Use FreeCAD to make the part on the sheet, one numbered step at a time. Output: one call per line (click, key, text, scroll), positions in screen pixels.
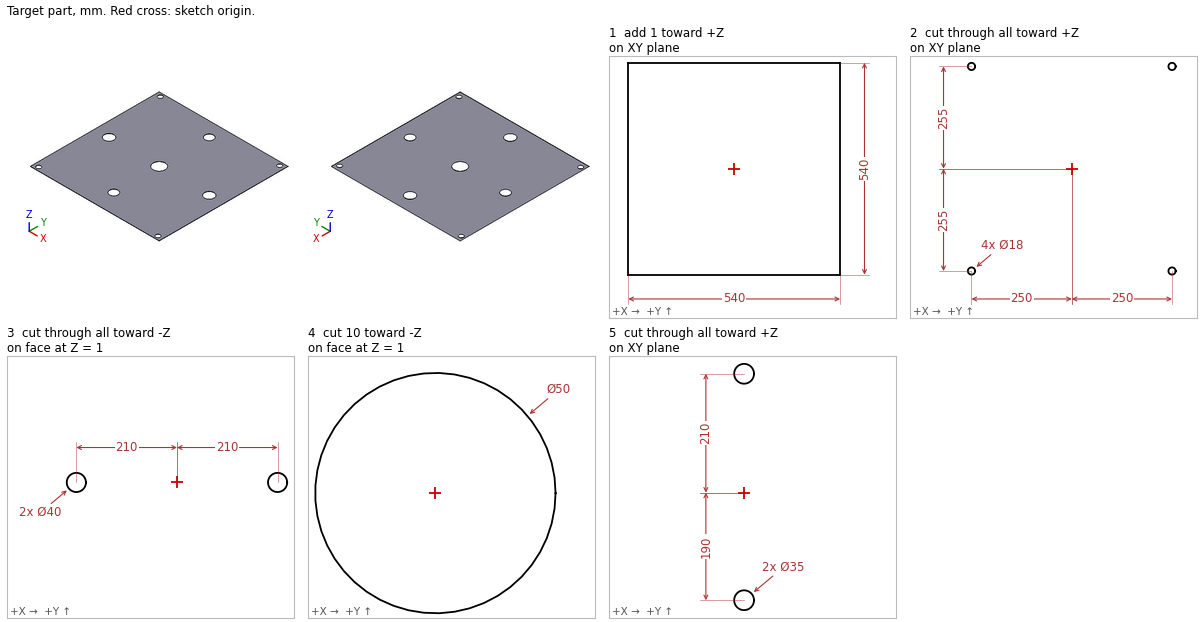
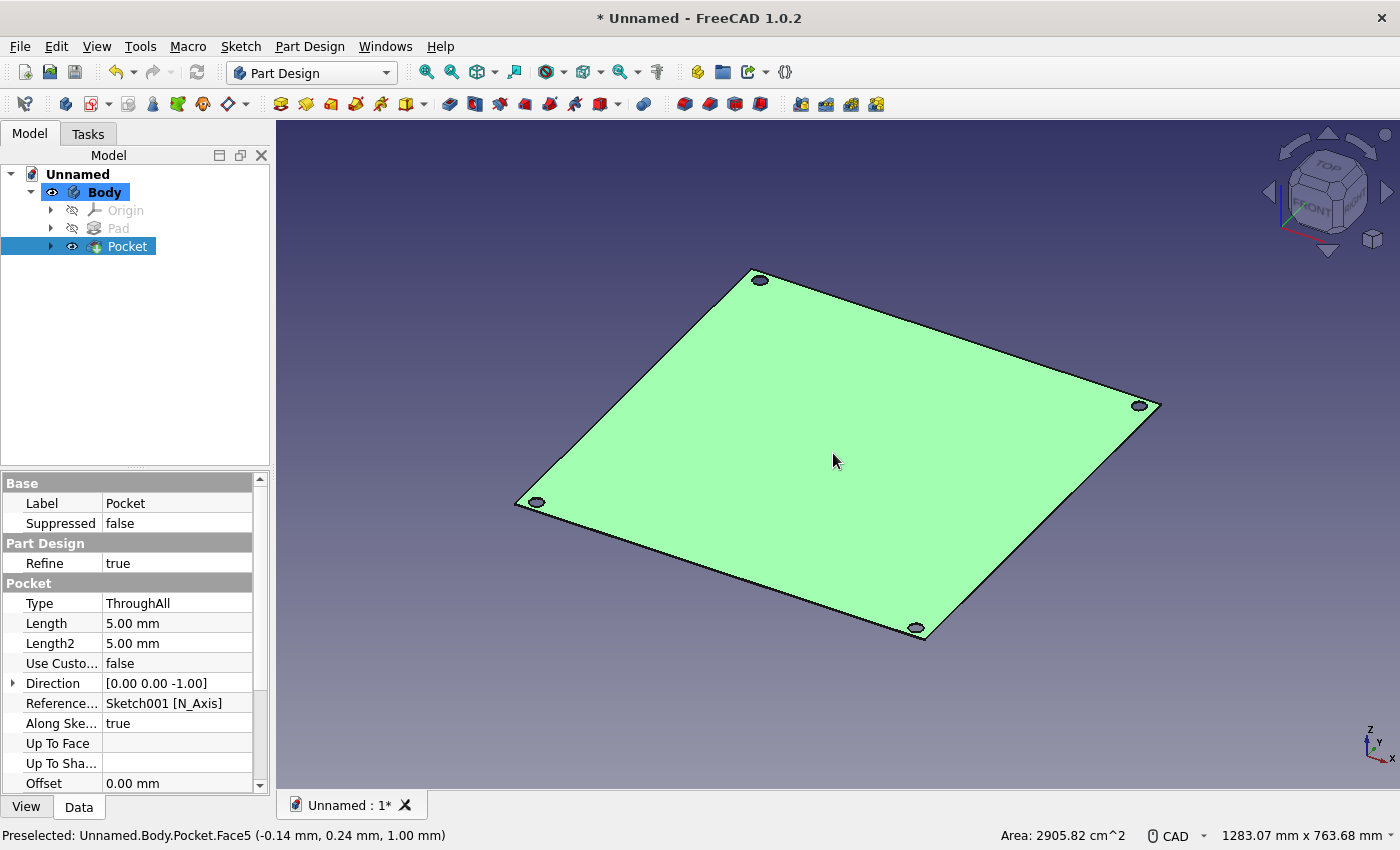
click(90, 104)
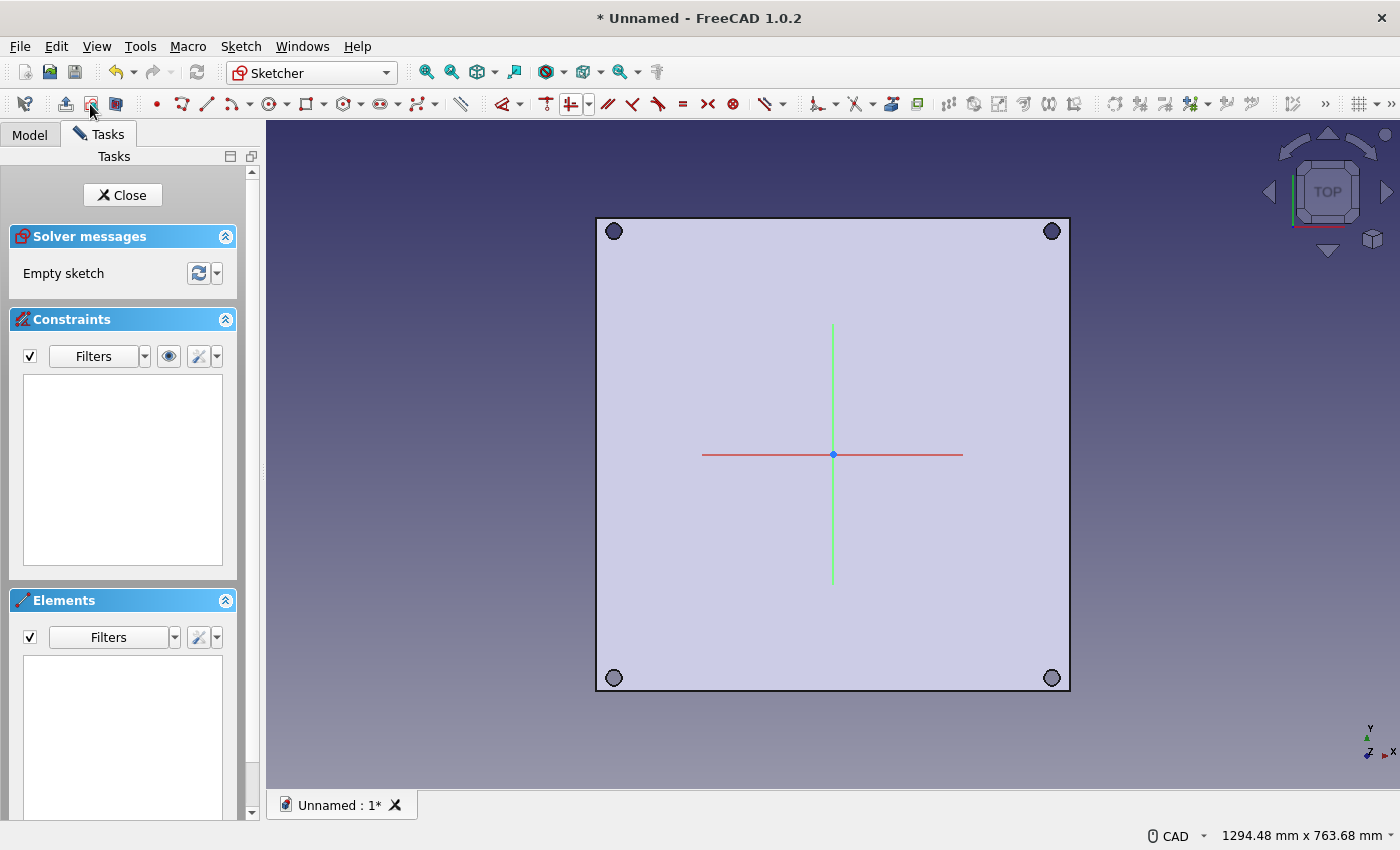
scroll(972, 455, up, 2)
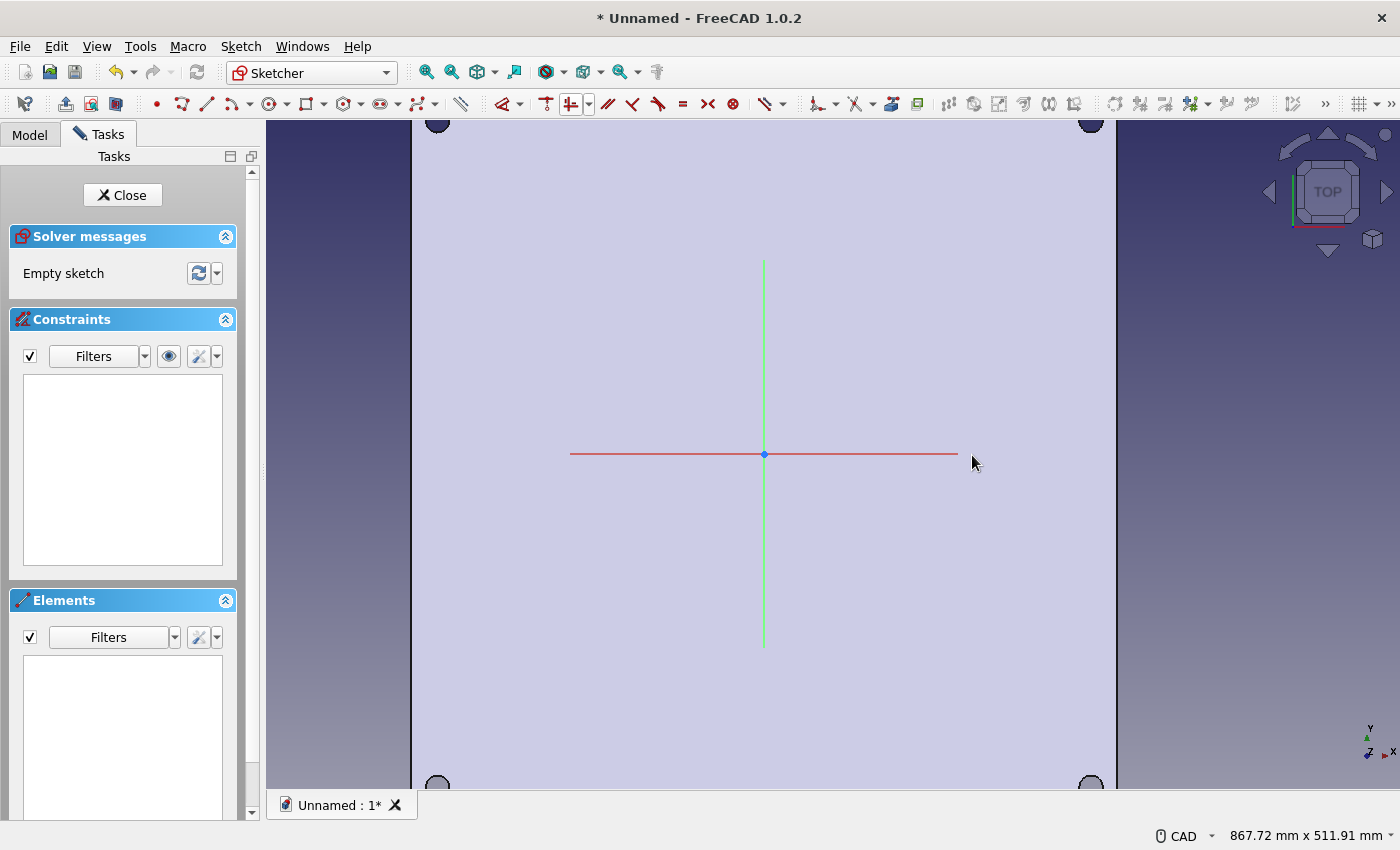
key(g)
key(c)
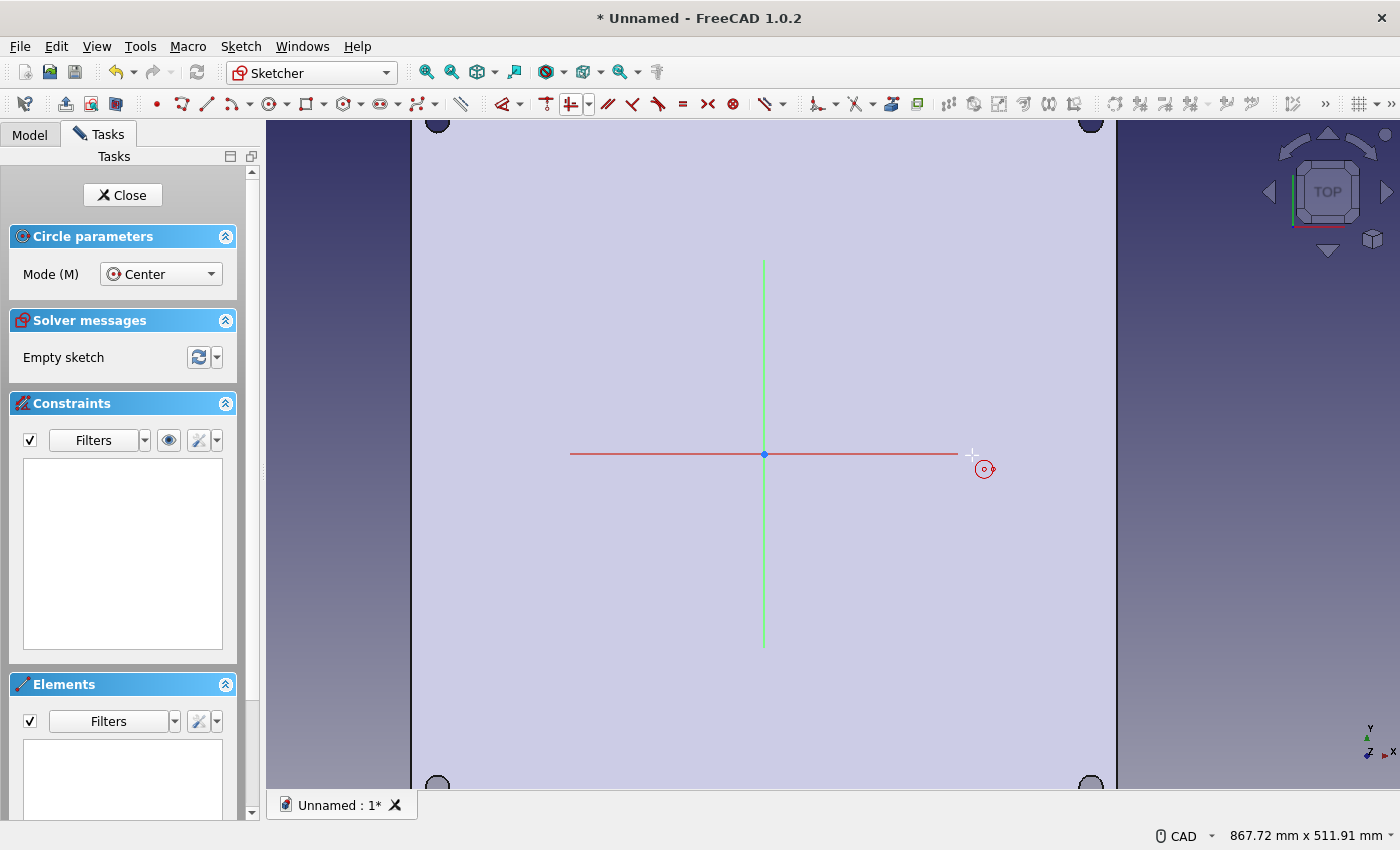
click(490, 454)
move(508, 436)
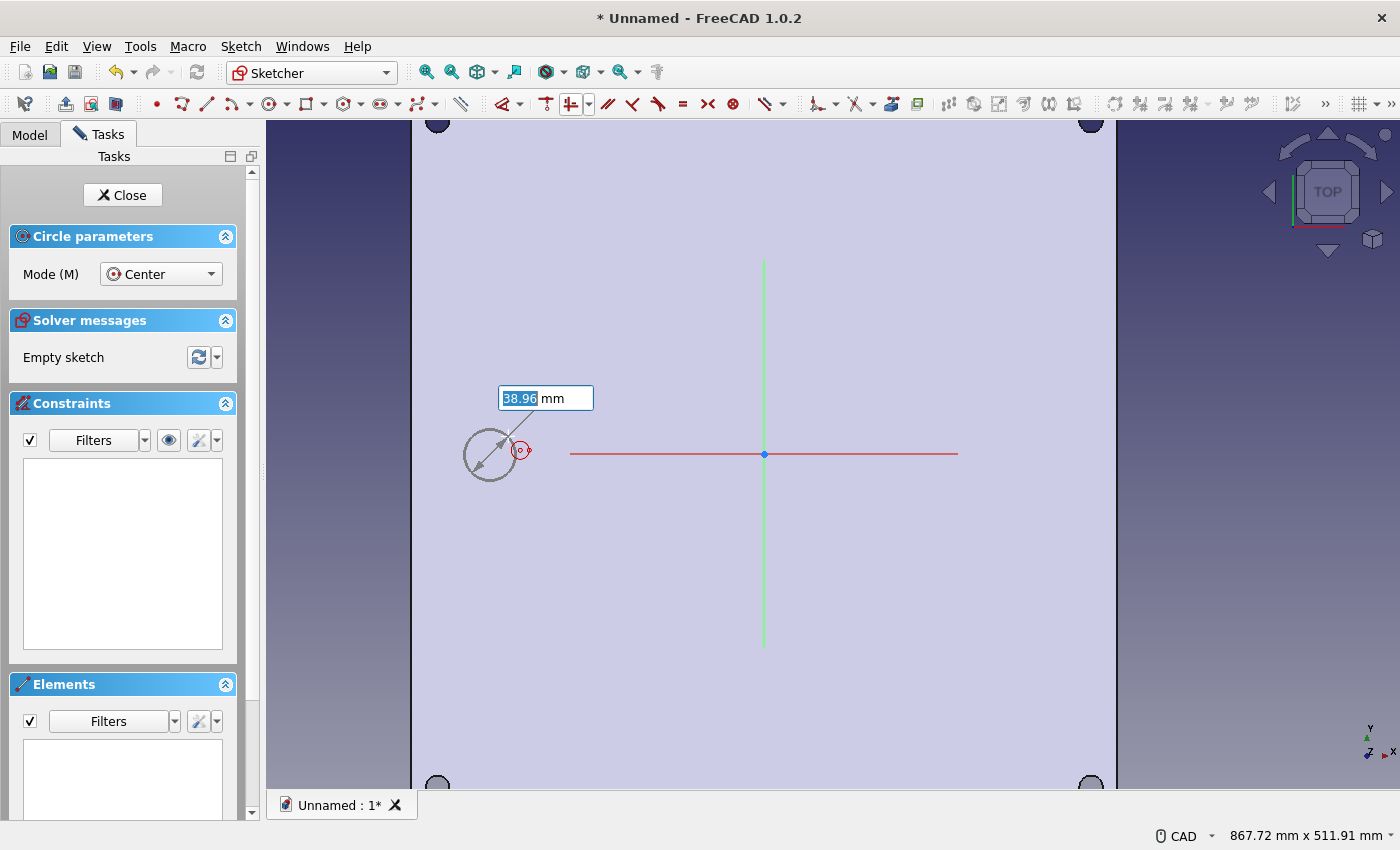
text(40)
key(Return)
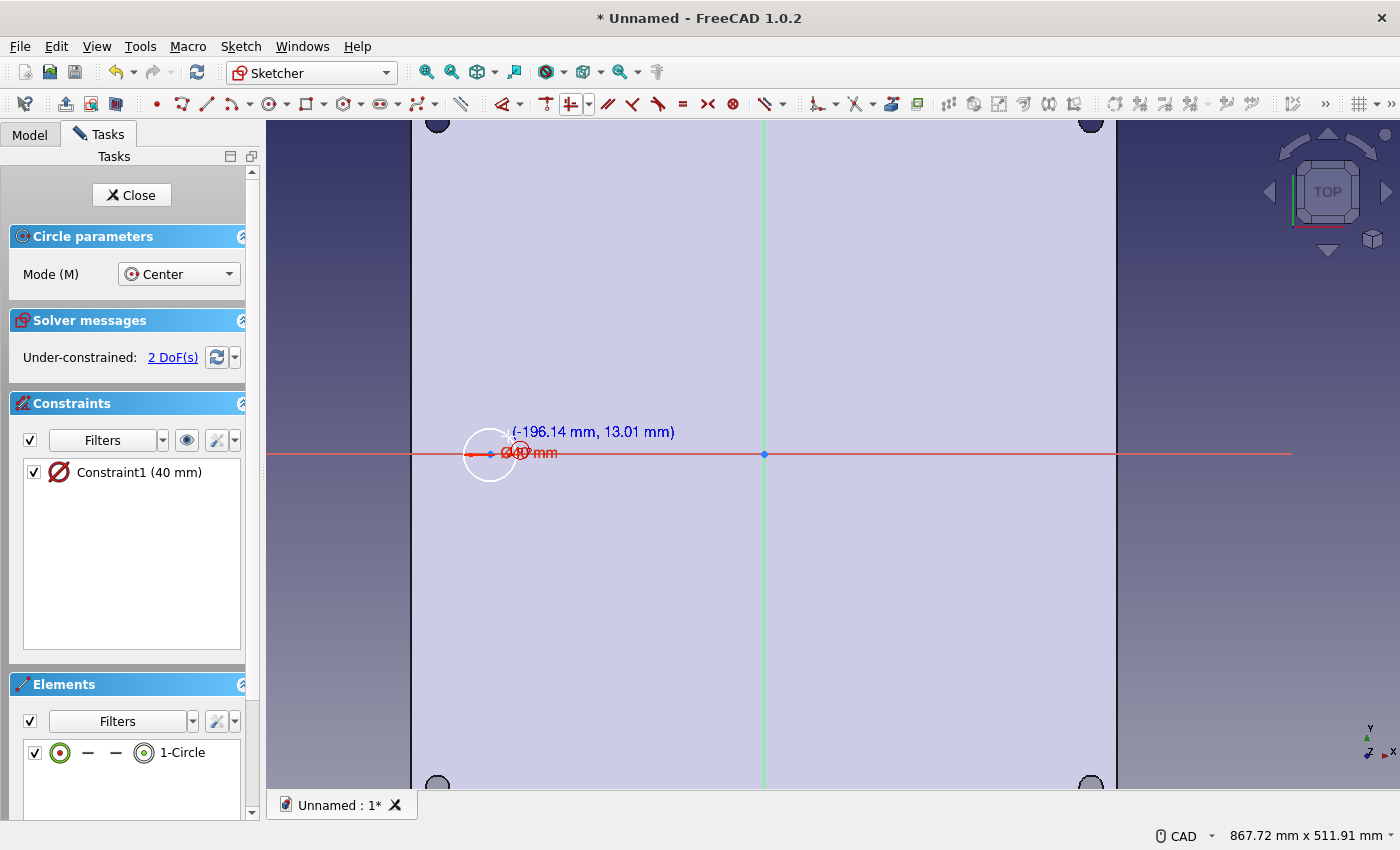
click(1039, 454)
move(1057, 436)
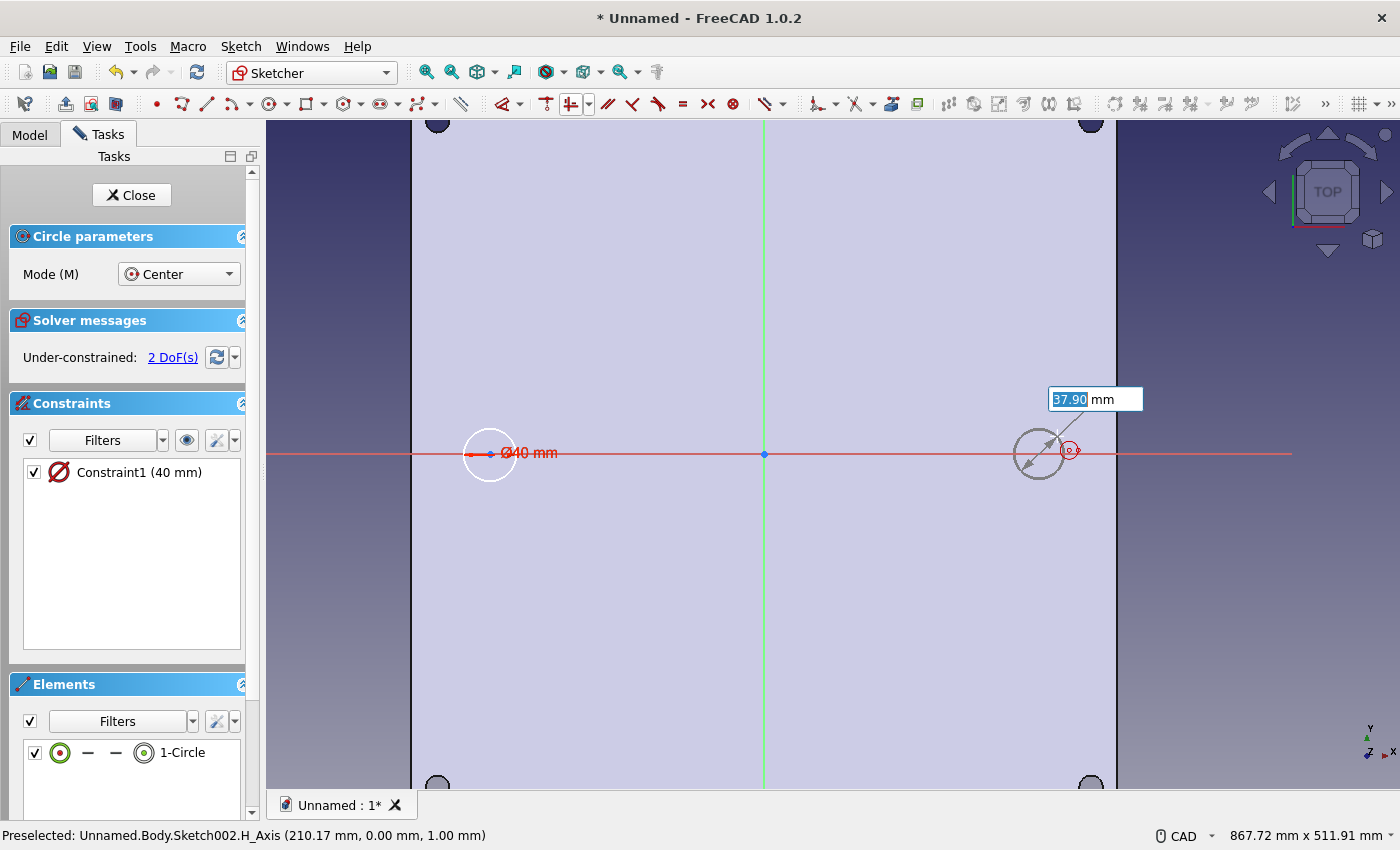
text(40)
key(Return)
key(Escape)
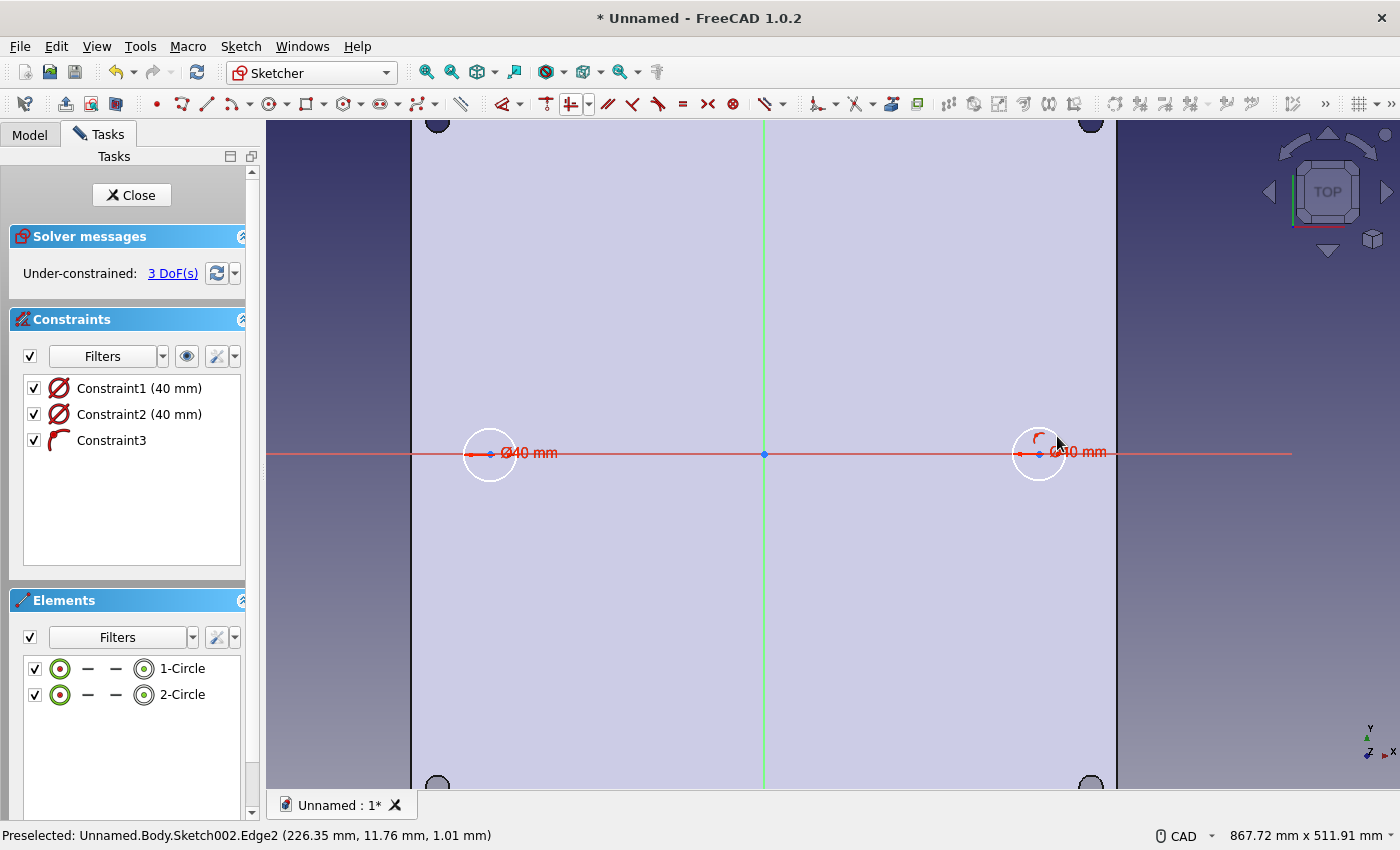
click(490, 455)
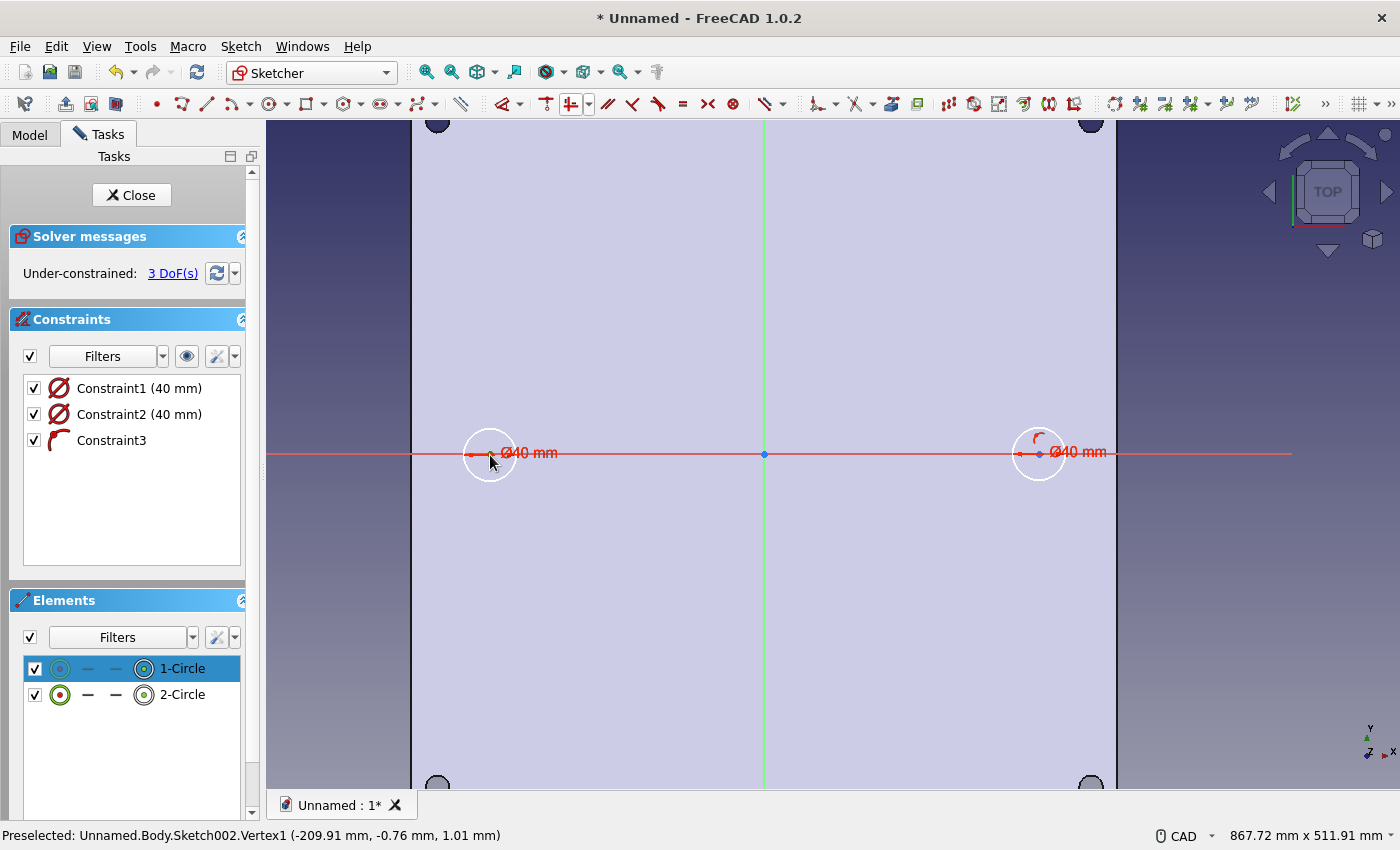
click(361, 454)